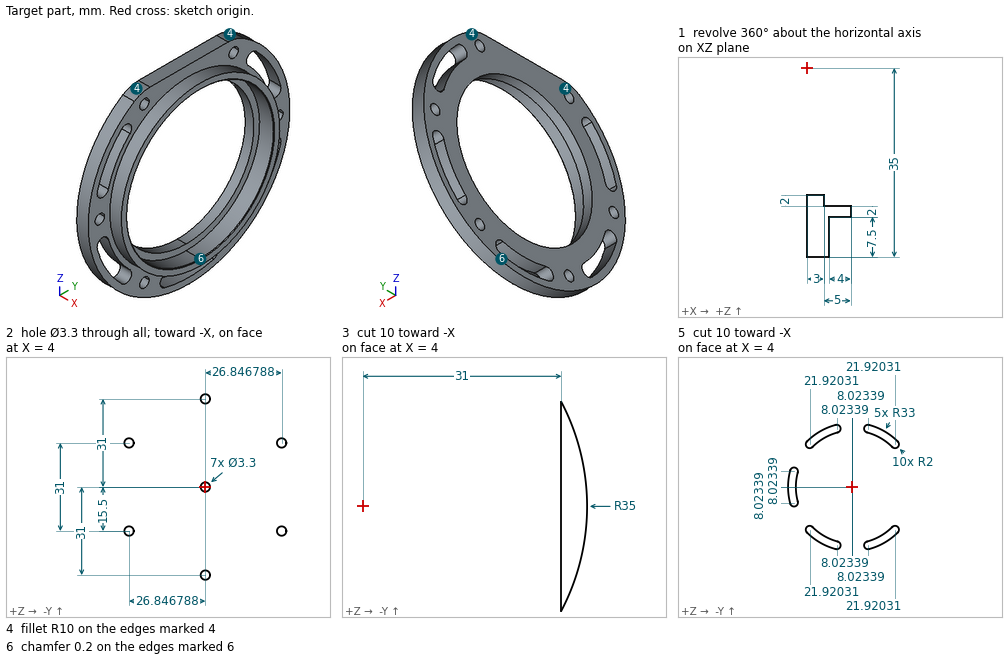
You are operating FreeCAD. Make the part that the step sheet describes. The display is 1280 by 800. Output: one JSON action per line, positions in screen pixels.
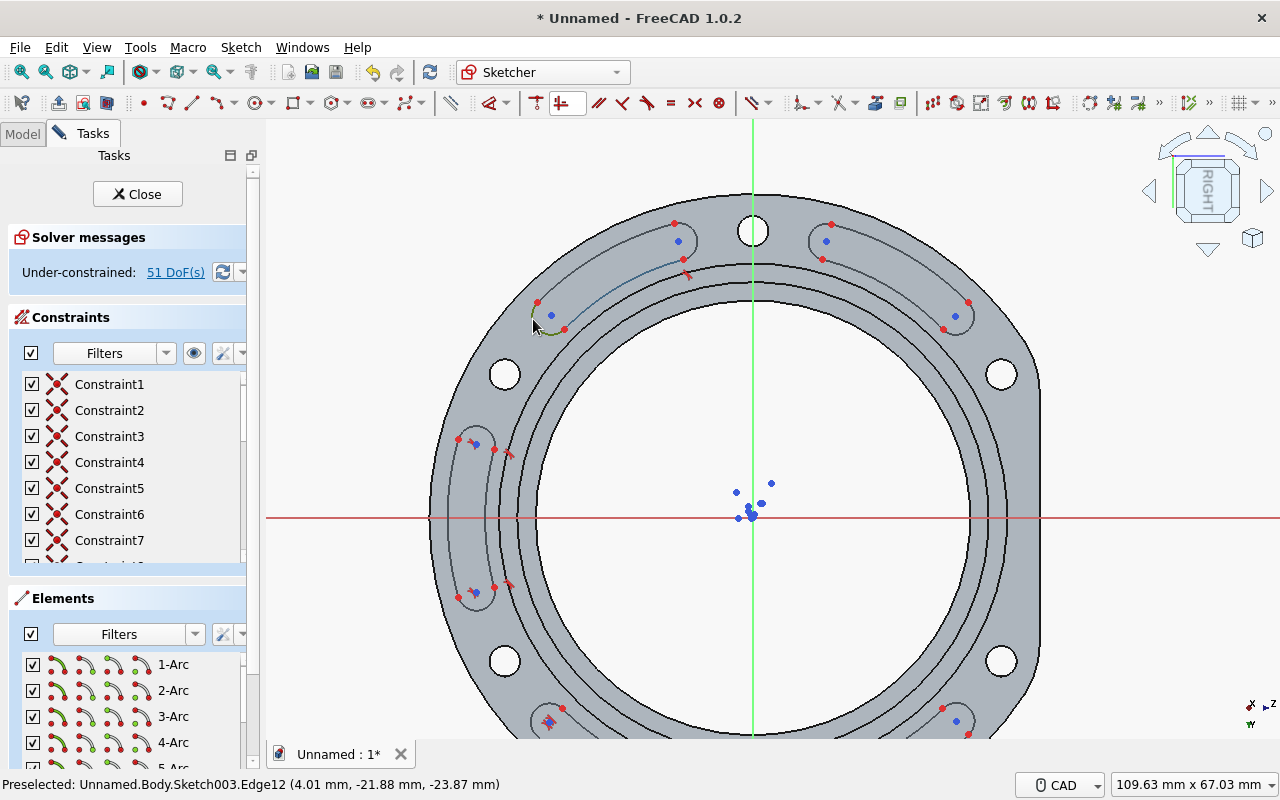
{"action": "left_click", "coordinate": [648, 104]}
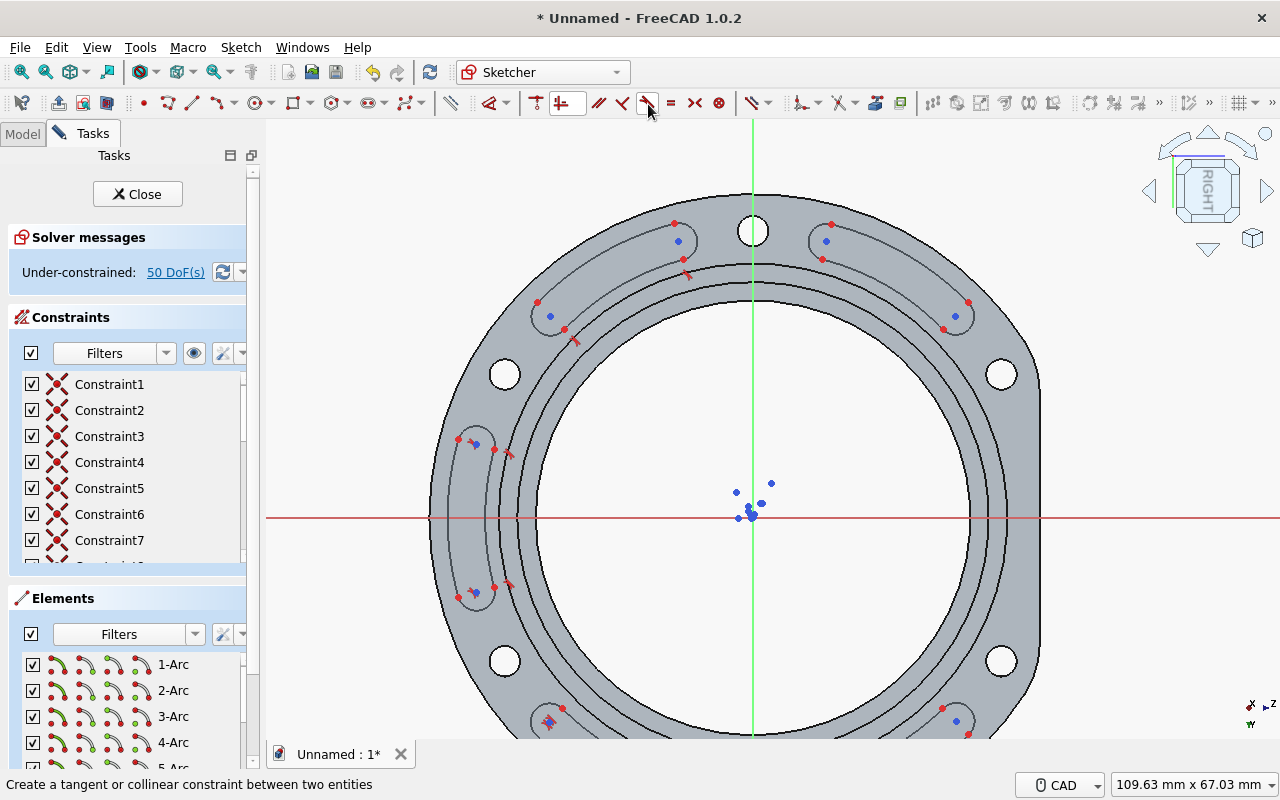
{"action": "left_click", "coordinate": [696, 248]}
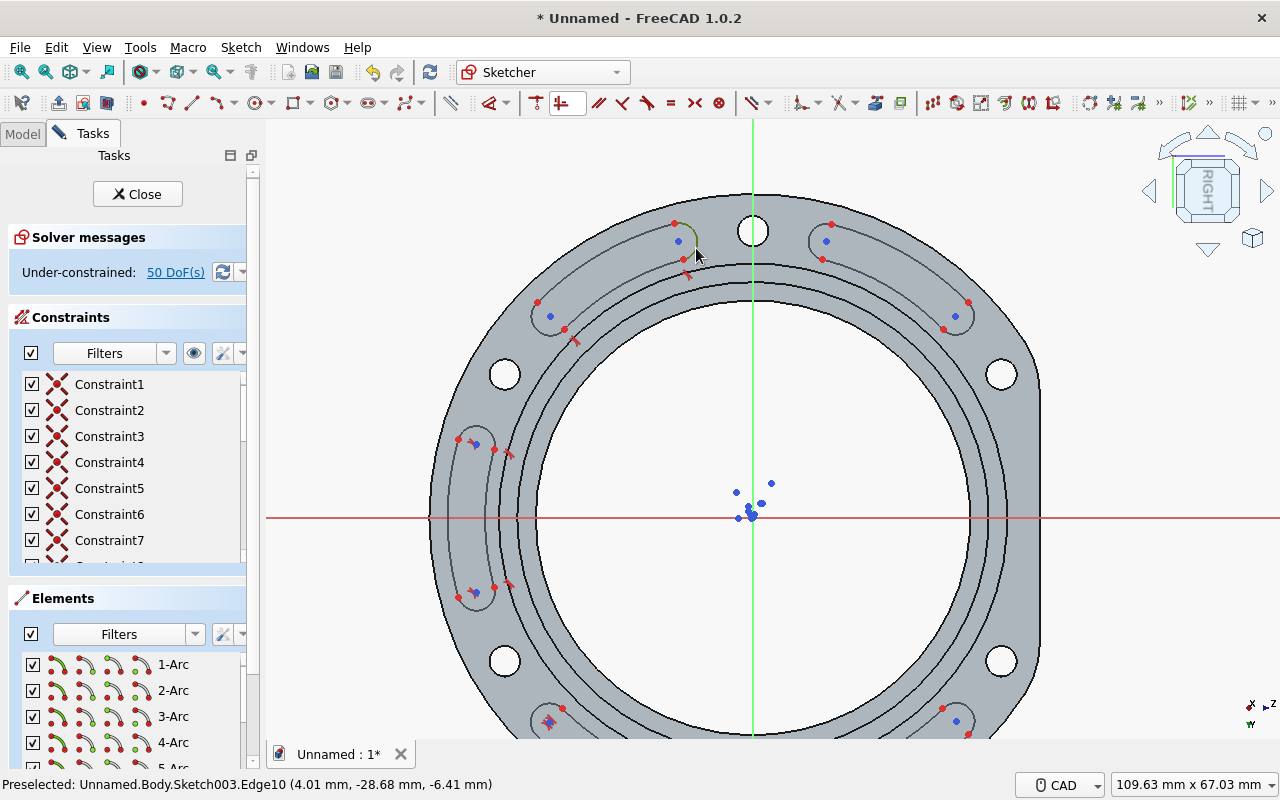
{"action": "left_click", "coordinate": [629, 240]}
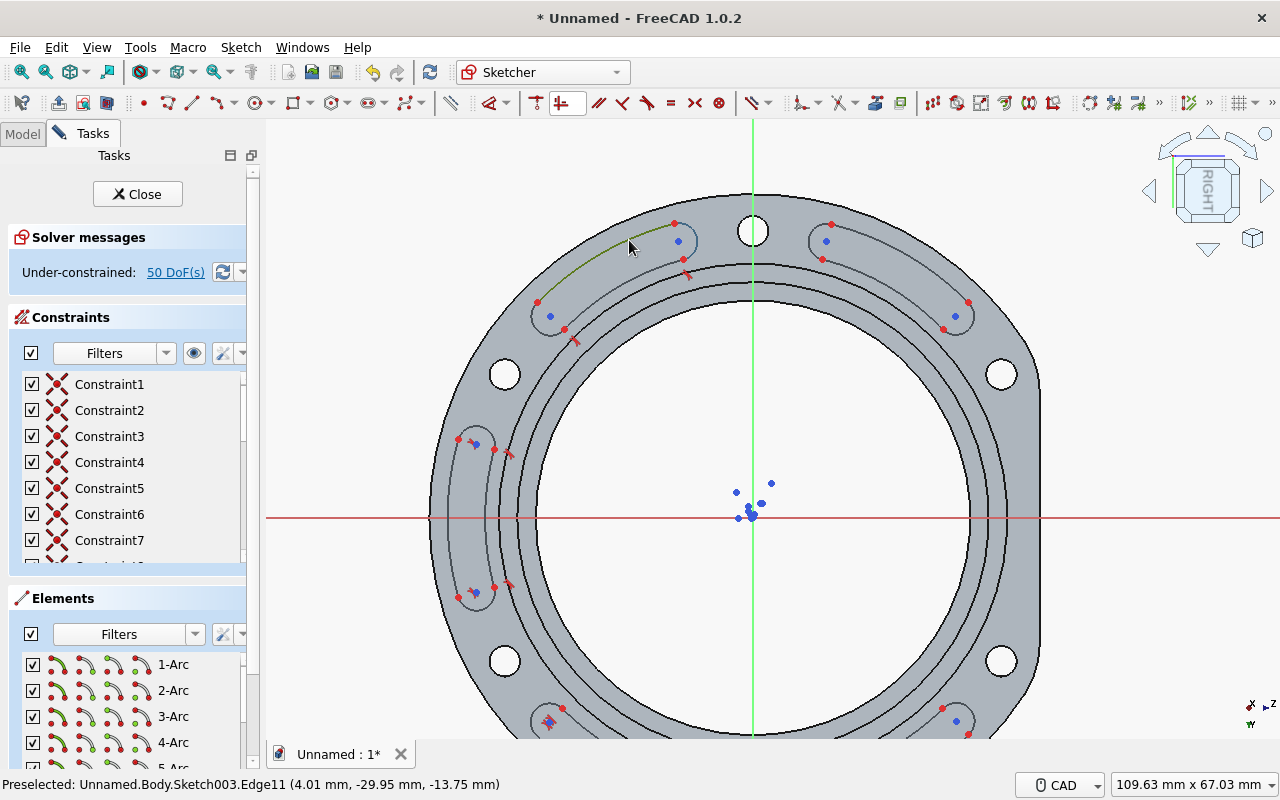
{"action": "left_click", "coordinate": [648, 104]}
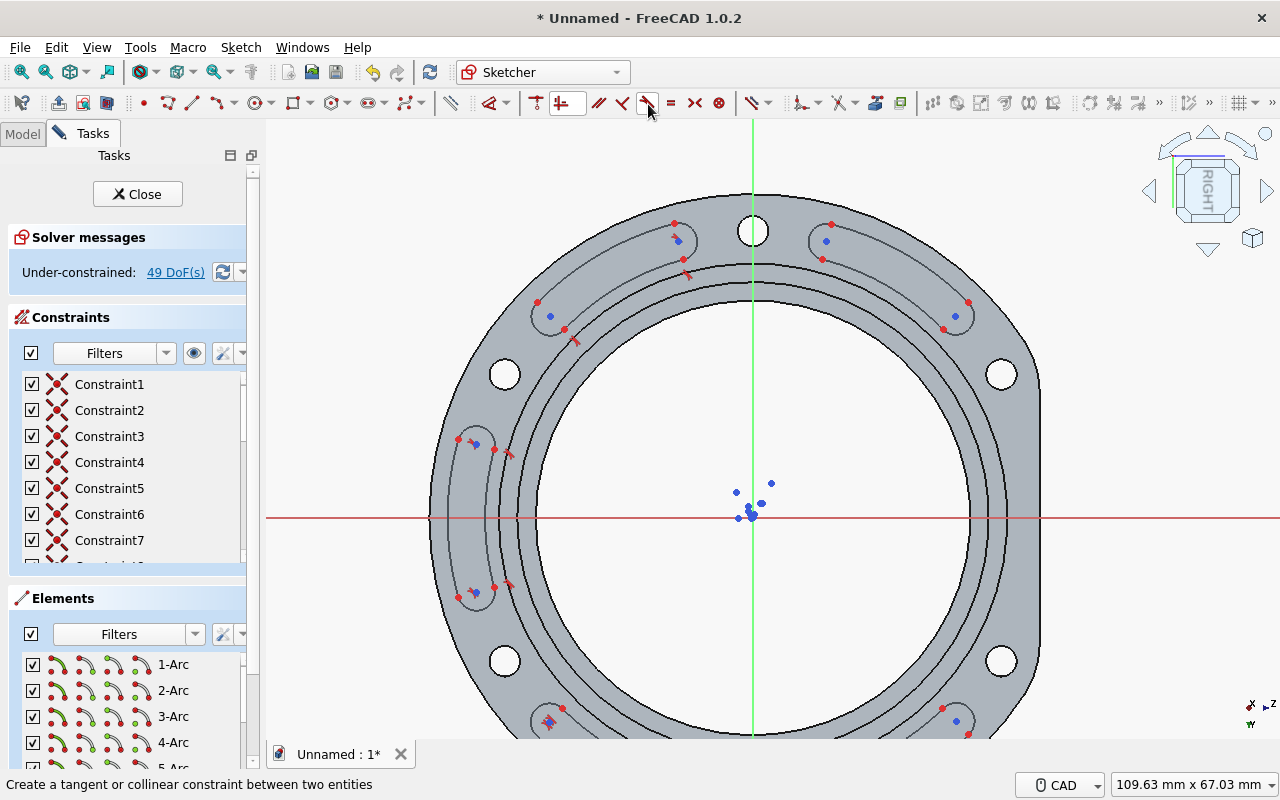
{"action": "left_click", "coordinate": [629, 240]}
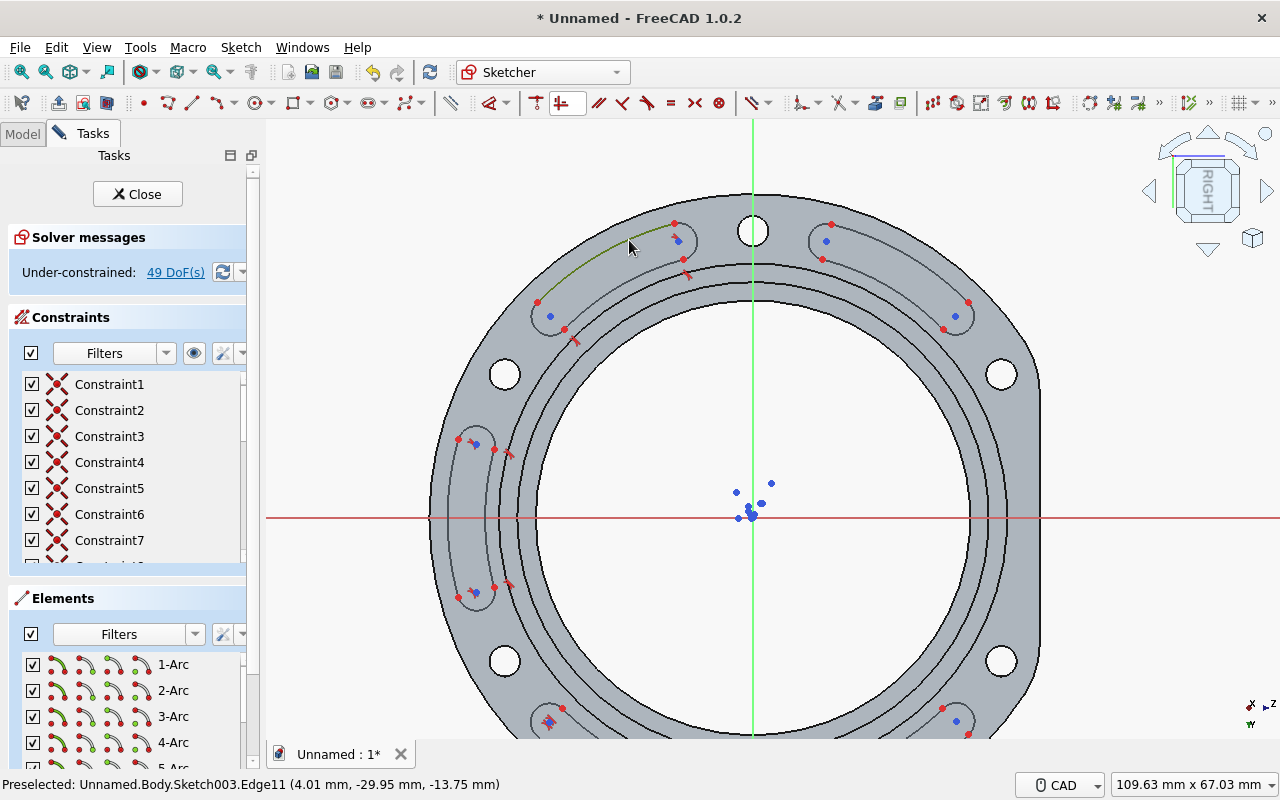
{"action": "left_click", "coordinate": [532, 319]}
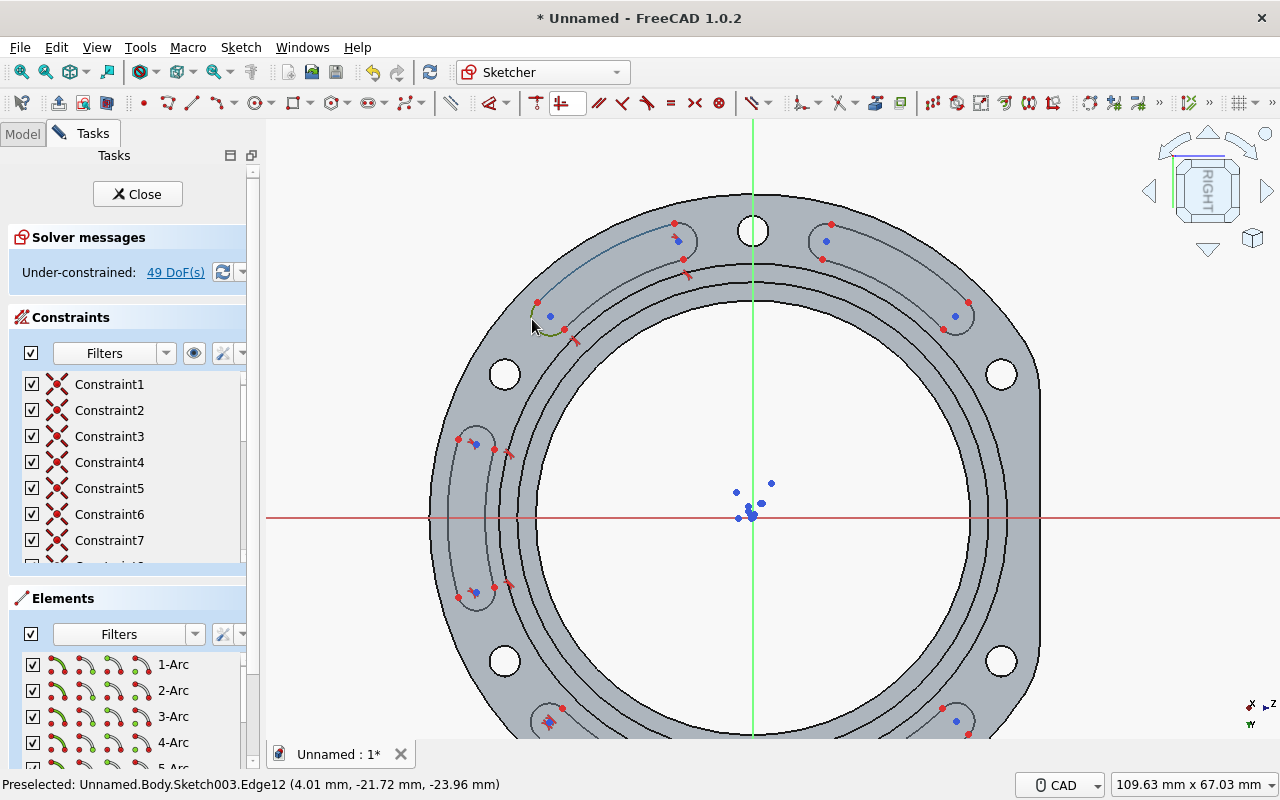
{"action": "left_click", "coordinate": [648, 104]}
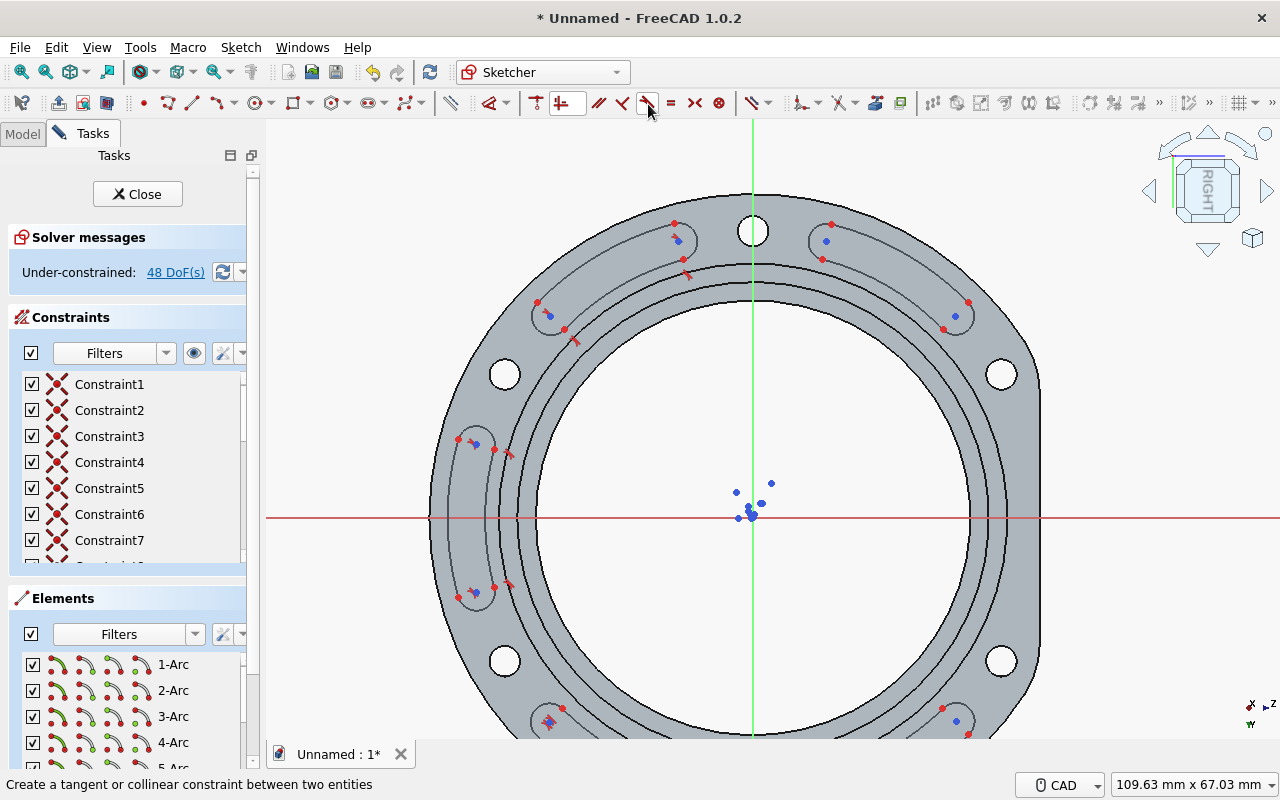
{"action": "left_click", "coordinate": [959, 334]}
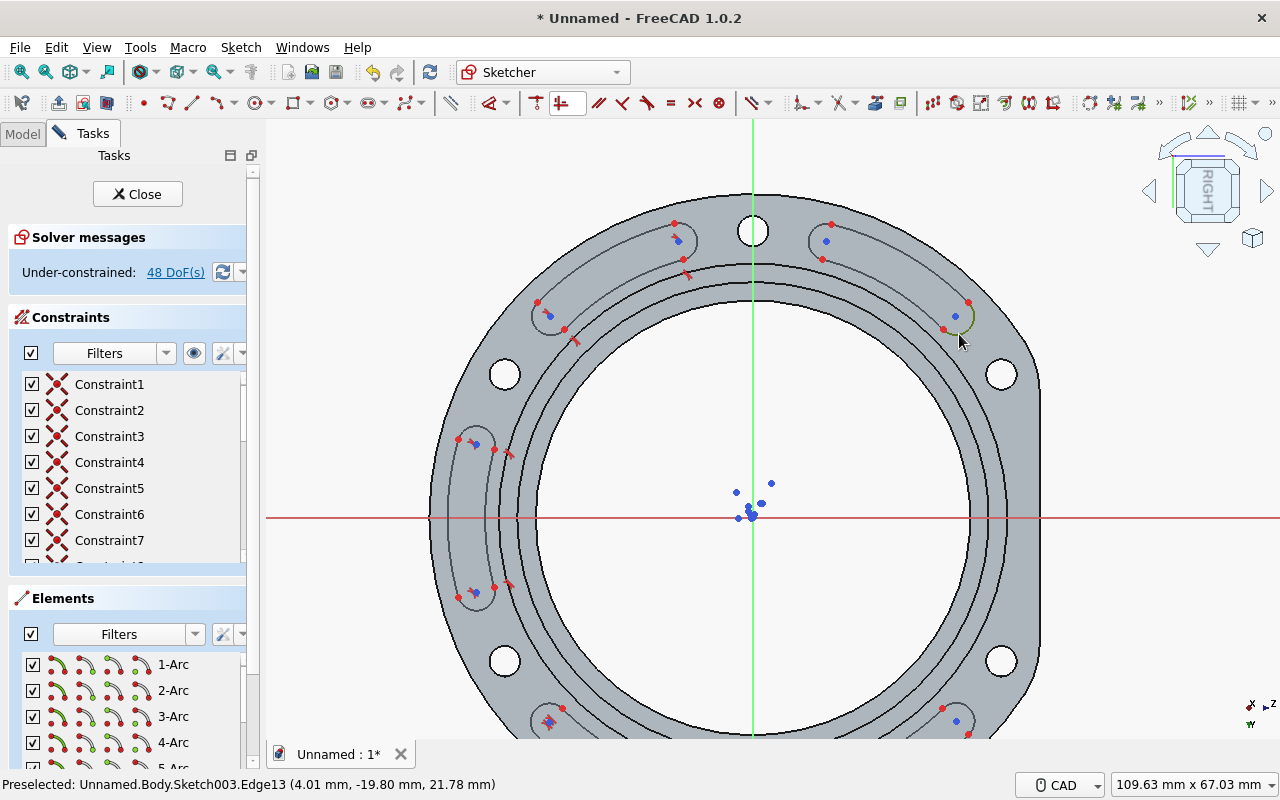
{"action": "left_click", "coordinate": [932, 272]}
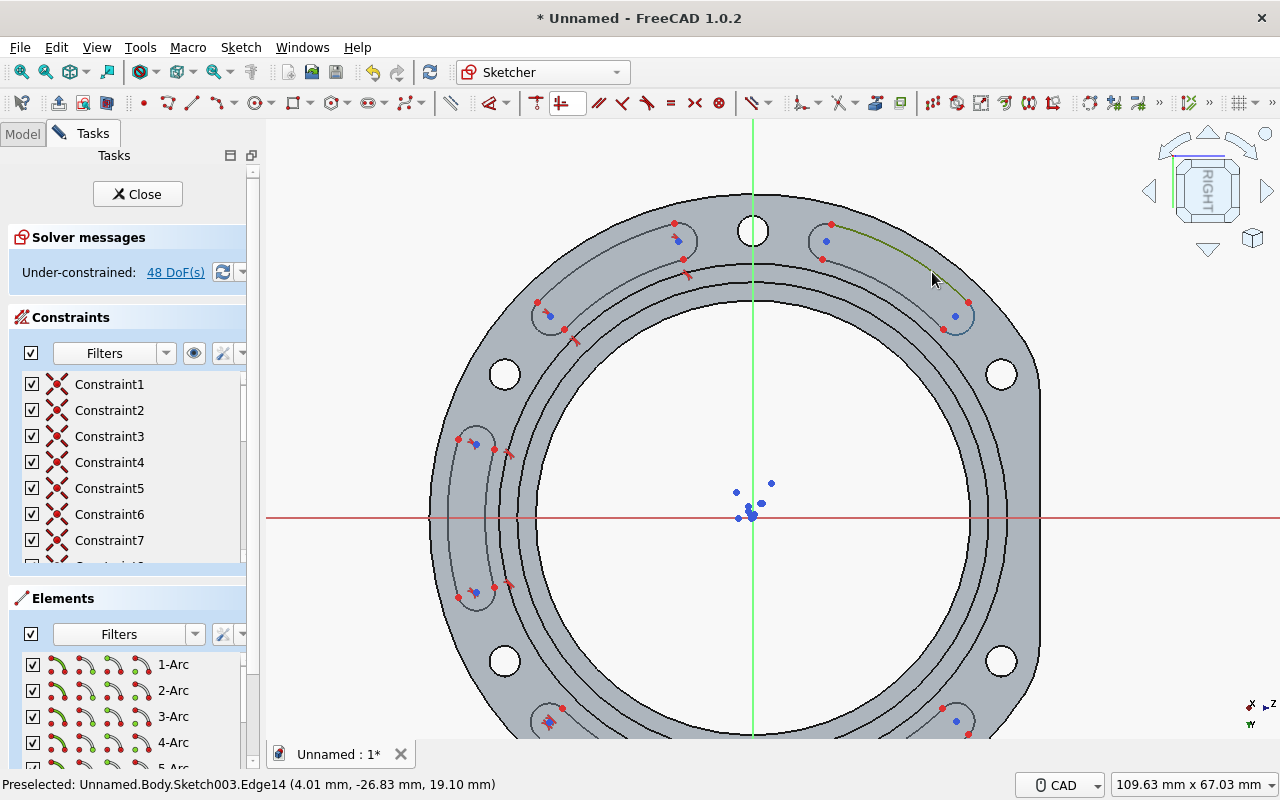
{"action": "left_click", "coordinate": [648, 104]}